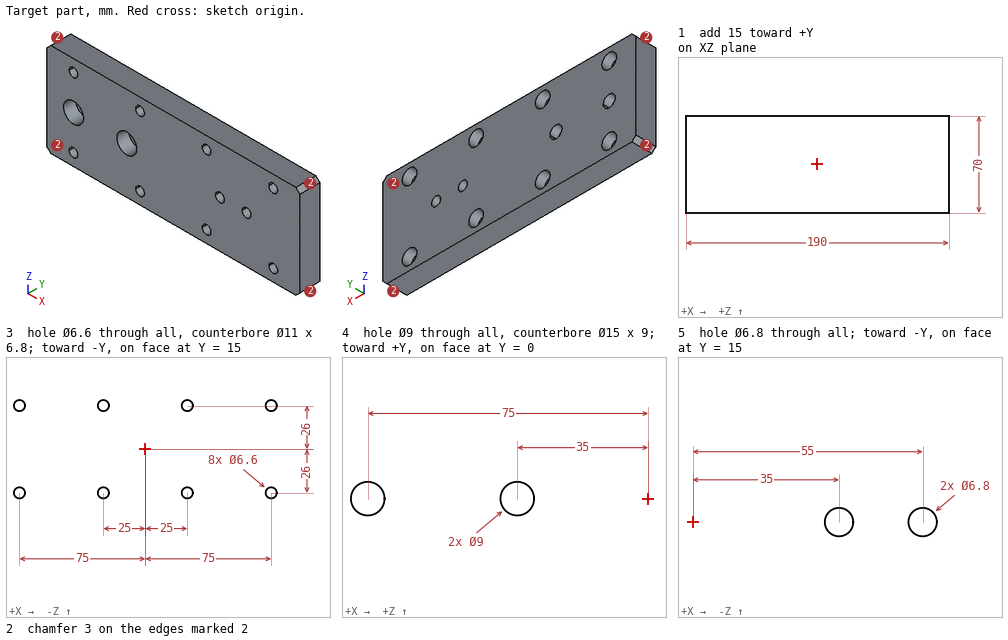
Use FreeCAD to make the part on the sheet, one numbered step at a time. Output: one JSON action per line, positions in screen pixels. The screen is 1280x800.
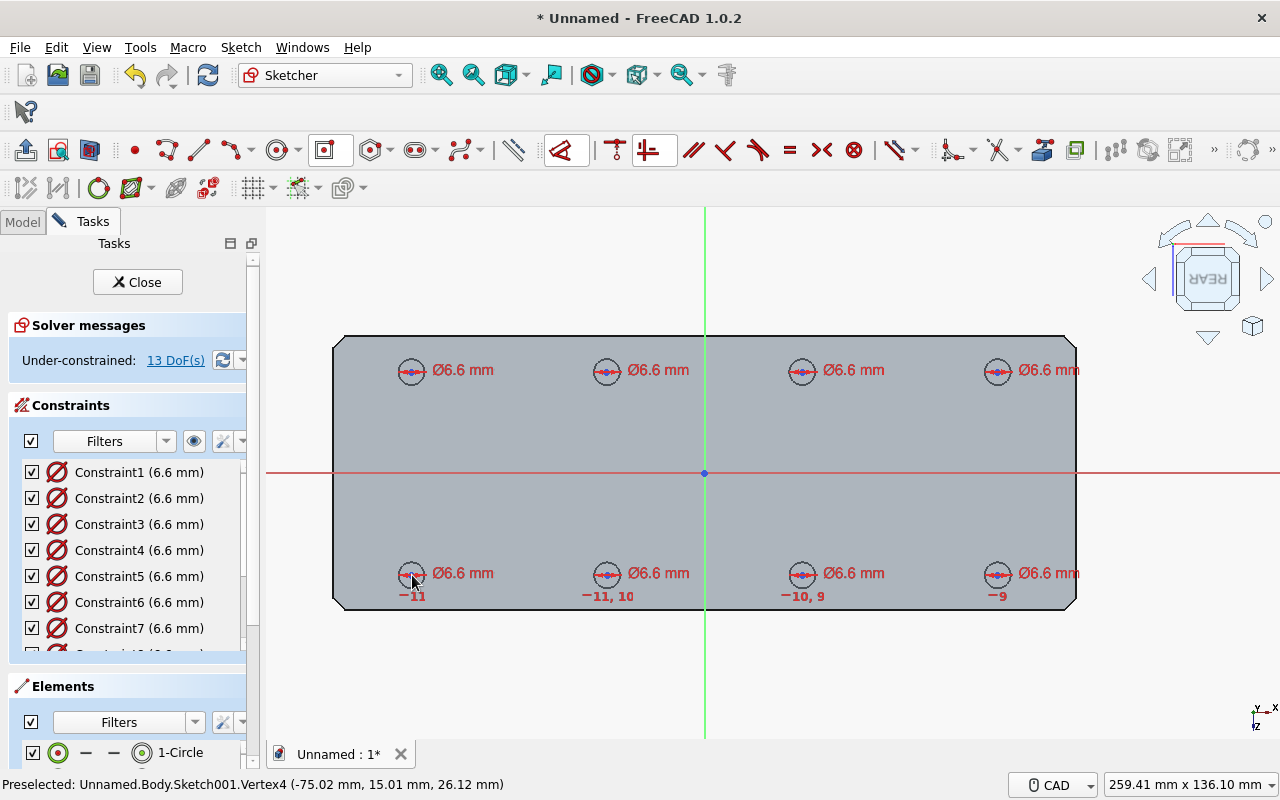
{"action": "left_click", "coordinate": [802, 575]}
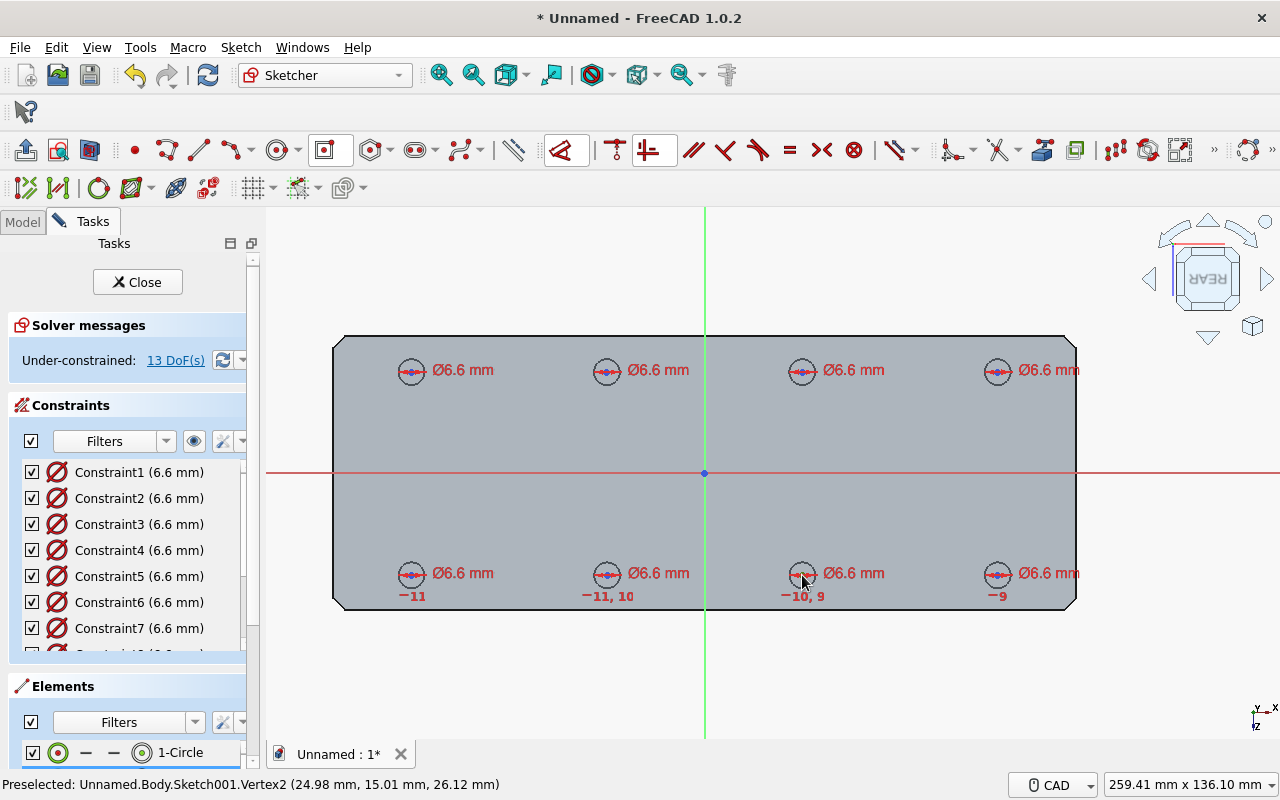
{"action": "left_click", "coordinate": [802, 372]}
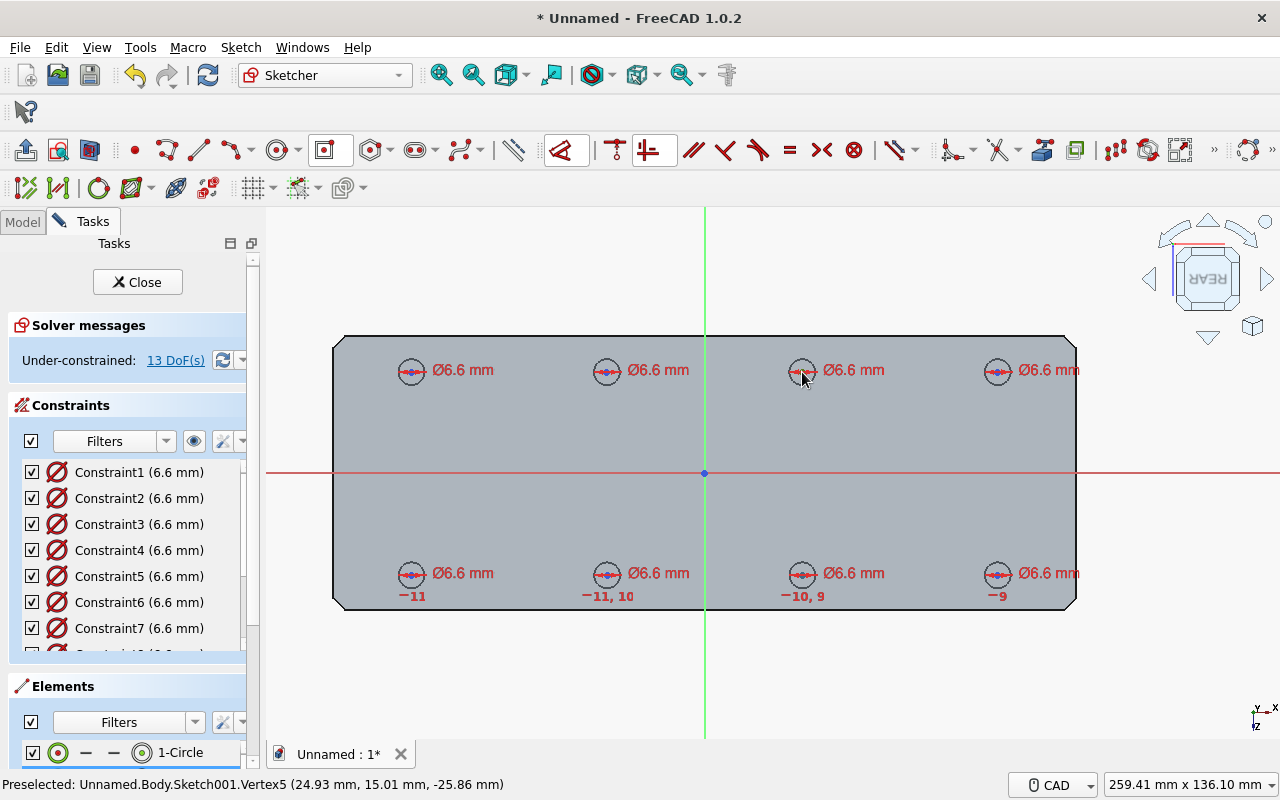
{"action": "key", "text": "v"}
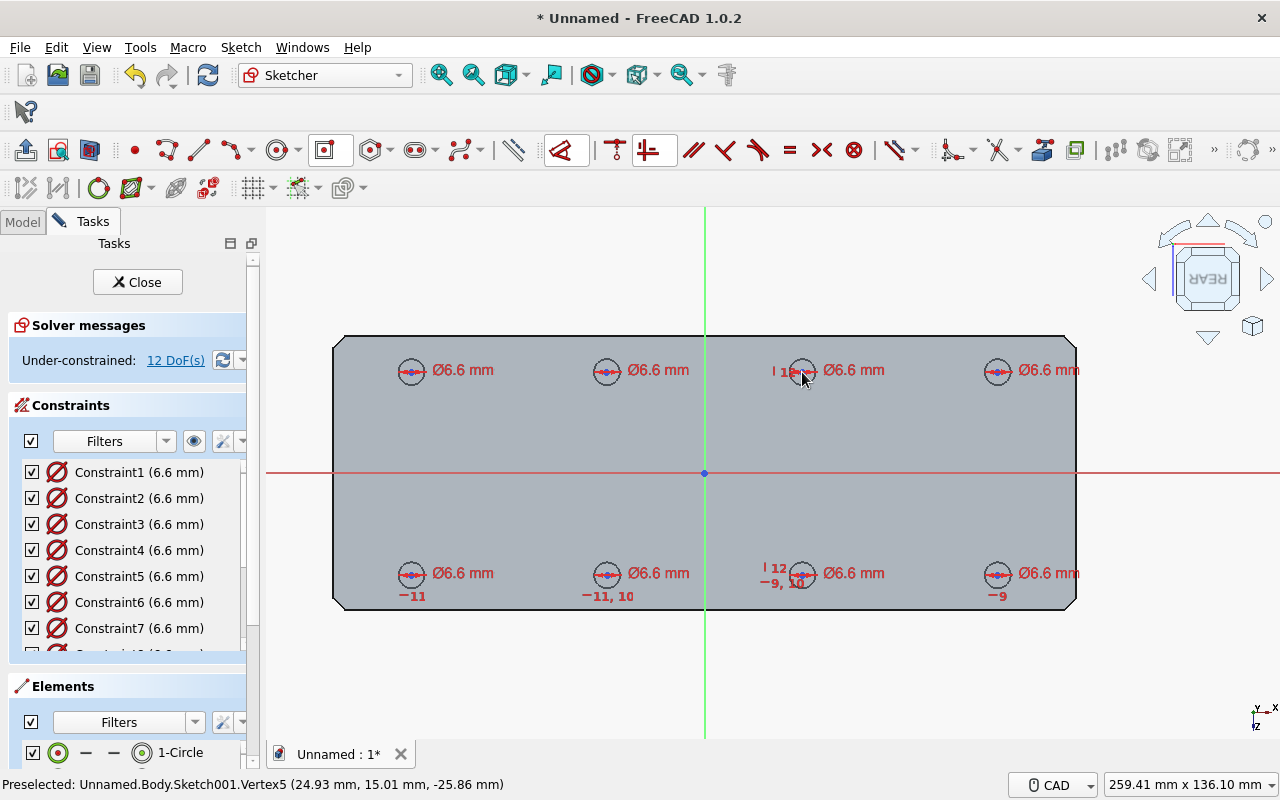
{"action": "left_click", "coordinate": [607, 575]}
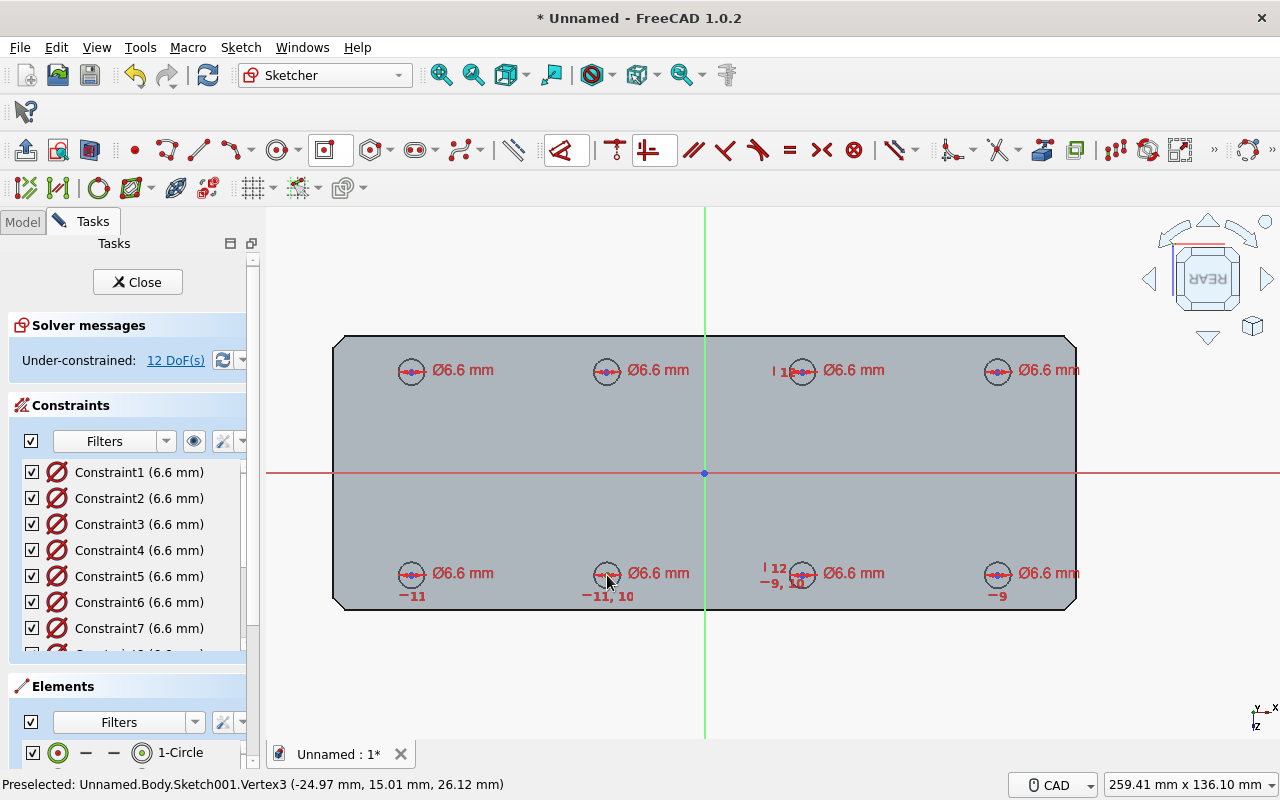
{"action": "left_click", "coordinate": [607, 372]}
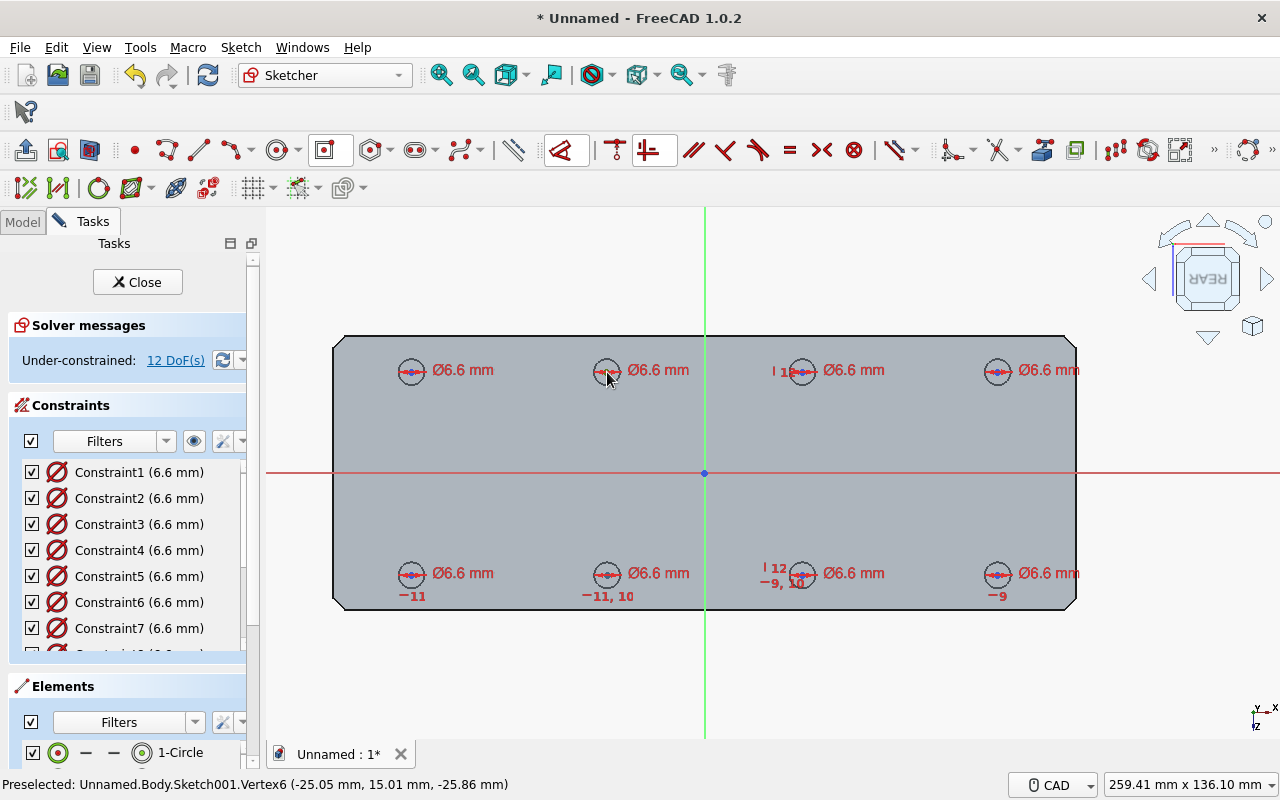
{"action": "key", "text": "v"}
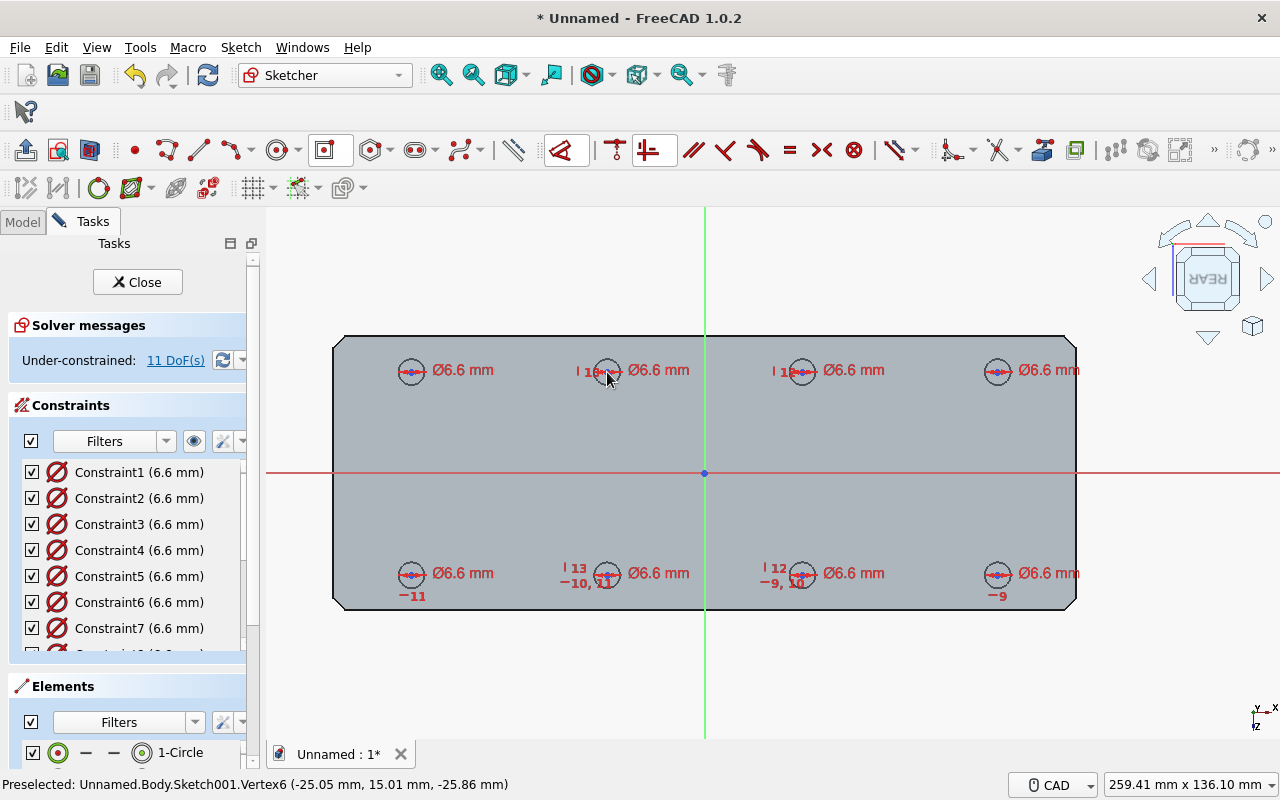
{"action": "left_click", "coordinate": [802, 372]}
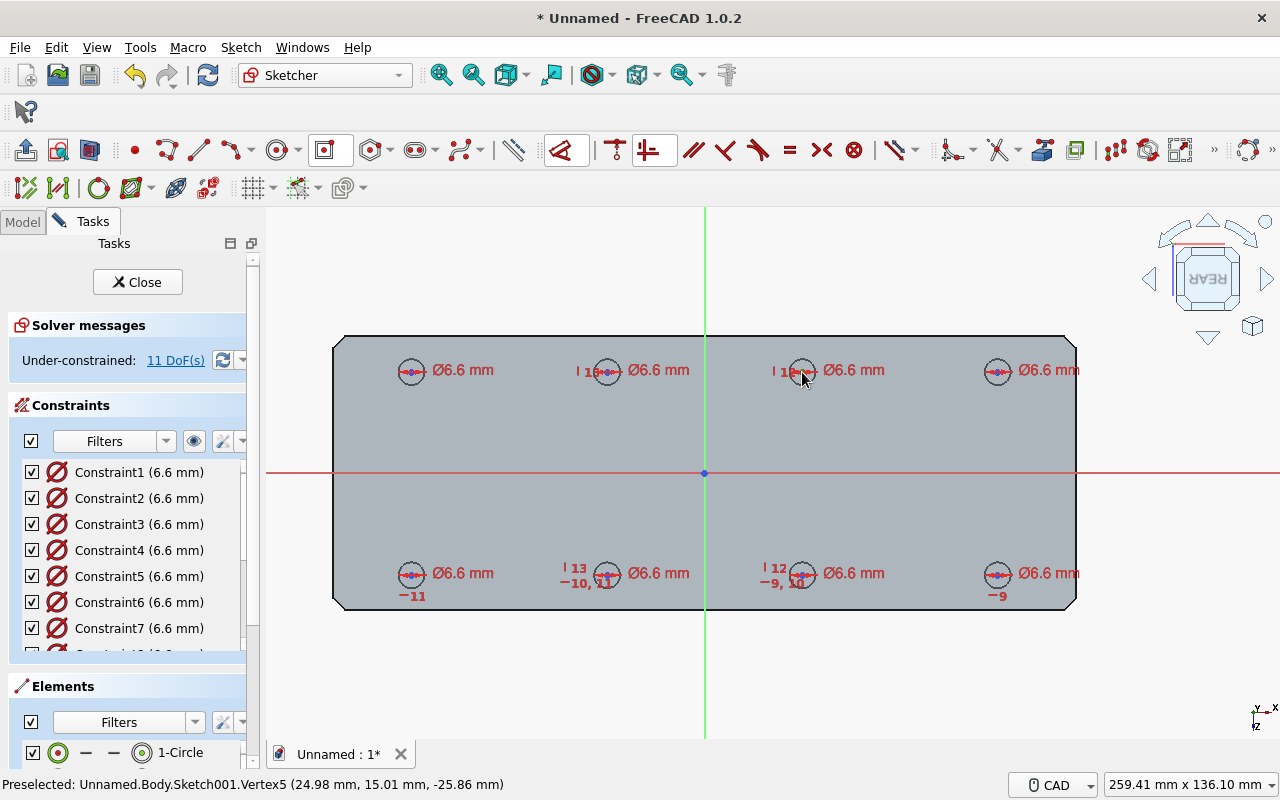
{"action": "left_click", "coordinate": [607, 372]}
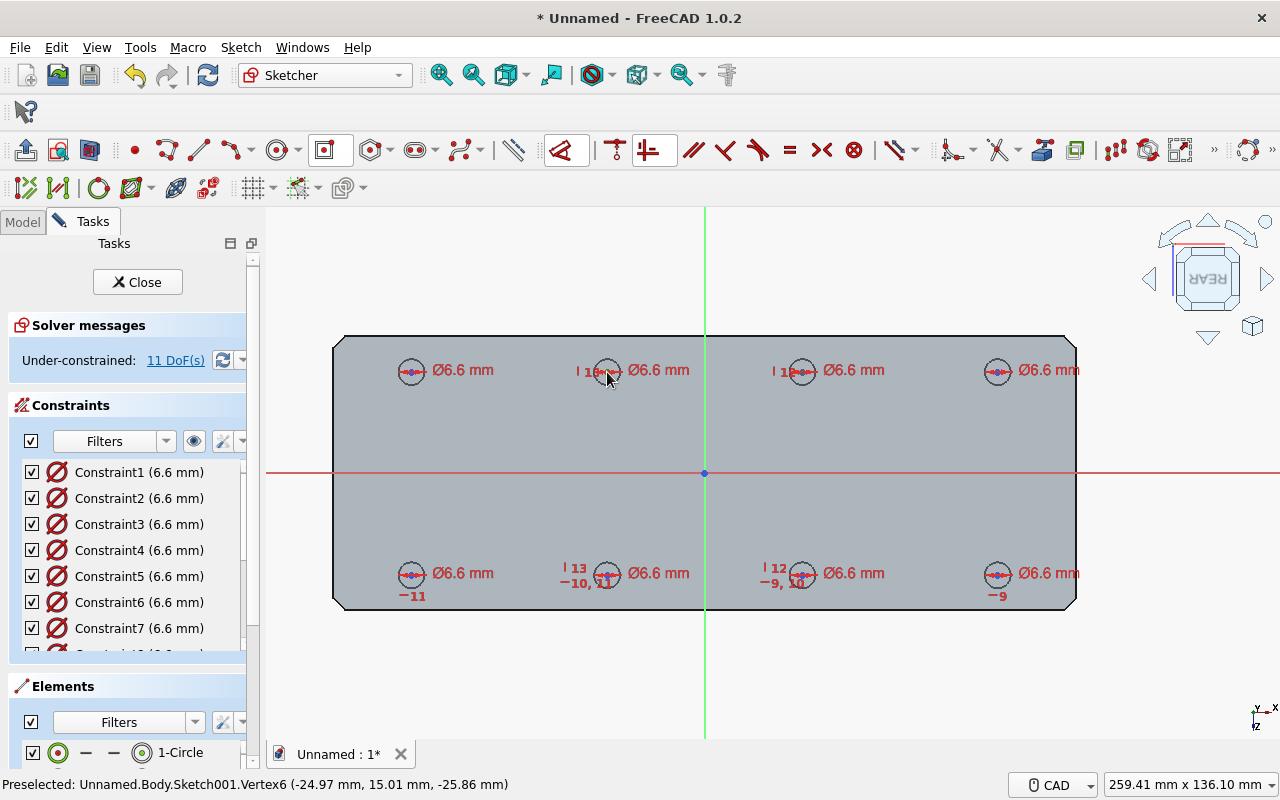
{"action": "left_click", "coordinate": [672, 150]}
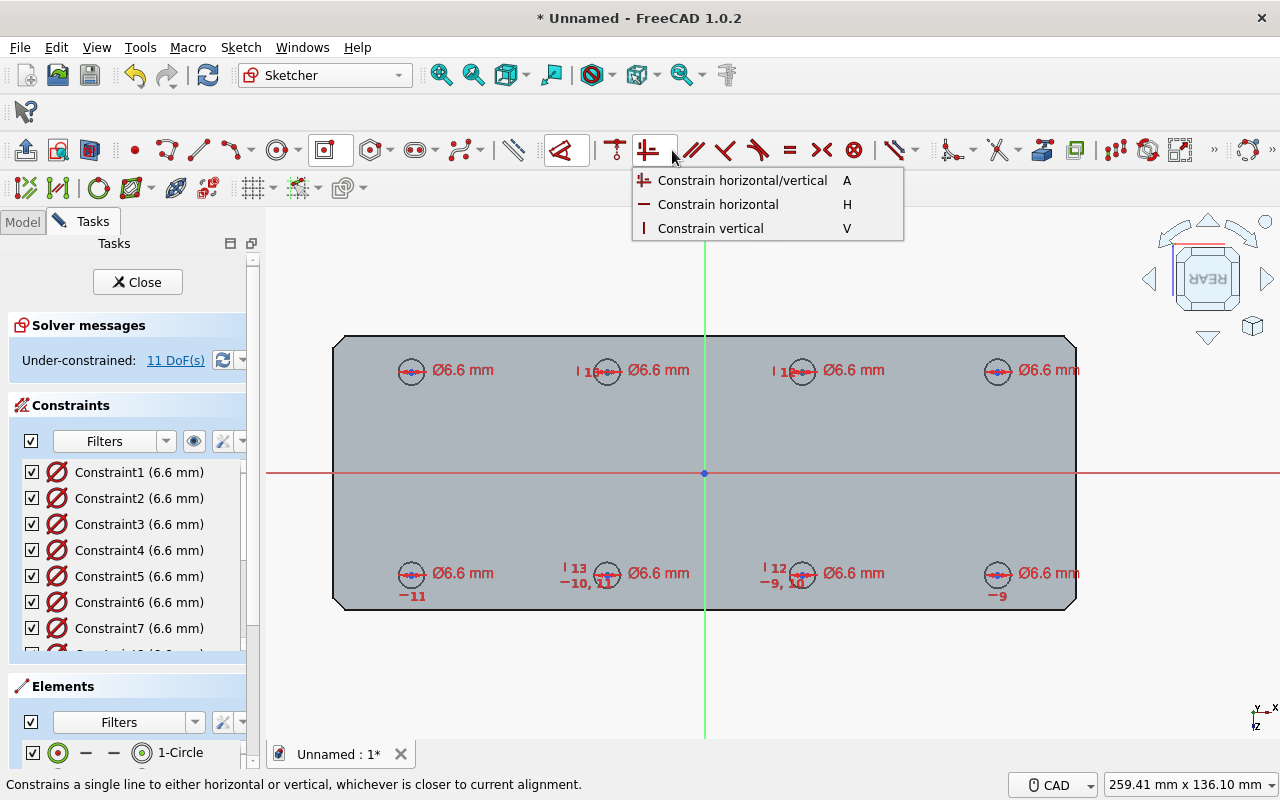
{"action": "left_click", "coordinate": [768, 204]}